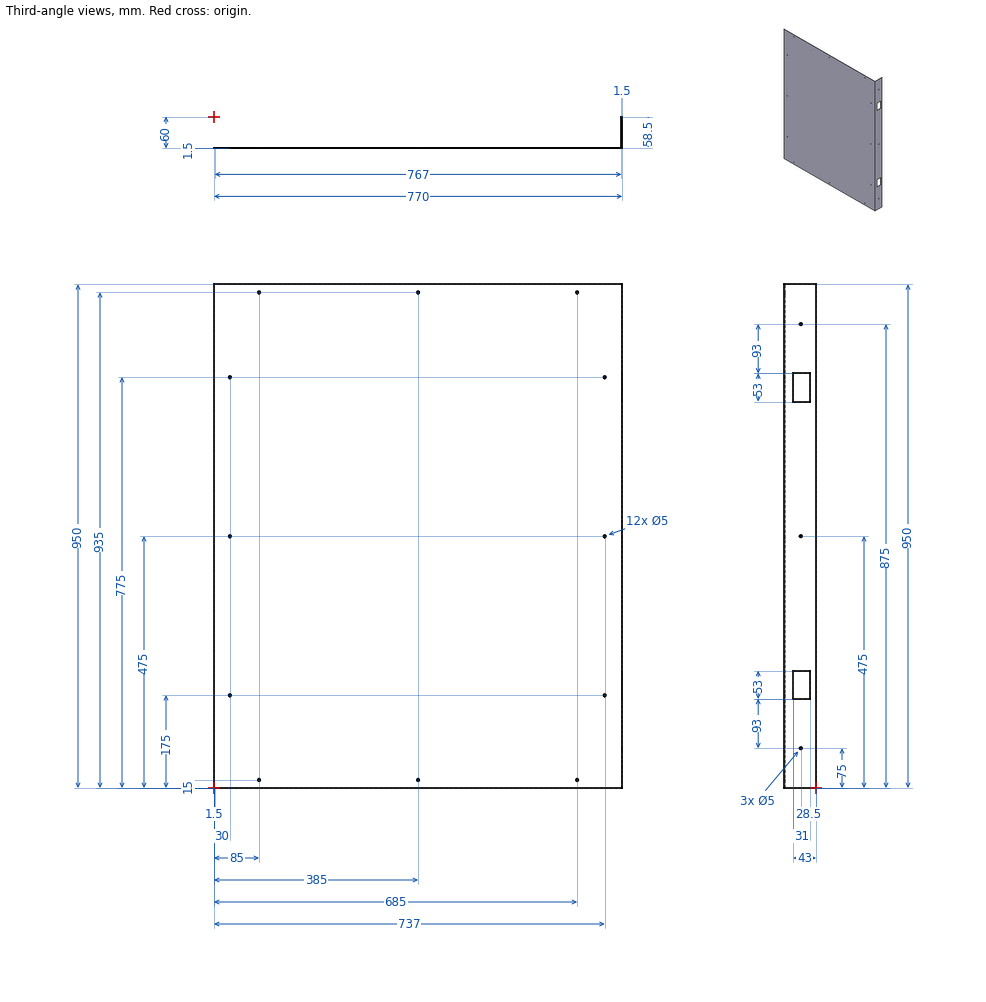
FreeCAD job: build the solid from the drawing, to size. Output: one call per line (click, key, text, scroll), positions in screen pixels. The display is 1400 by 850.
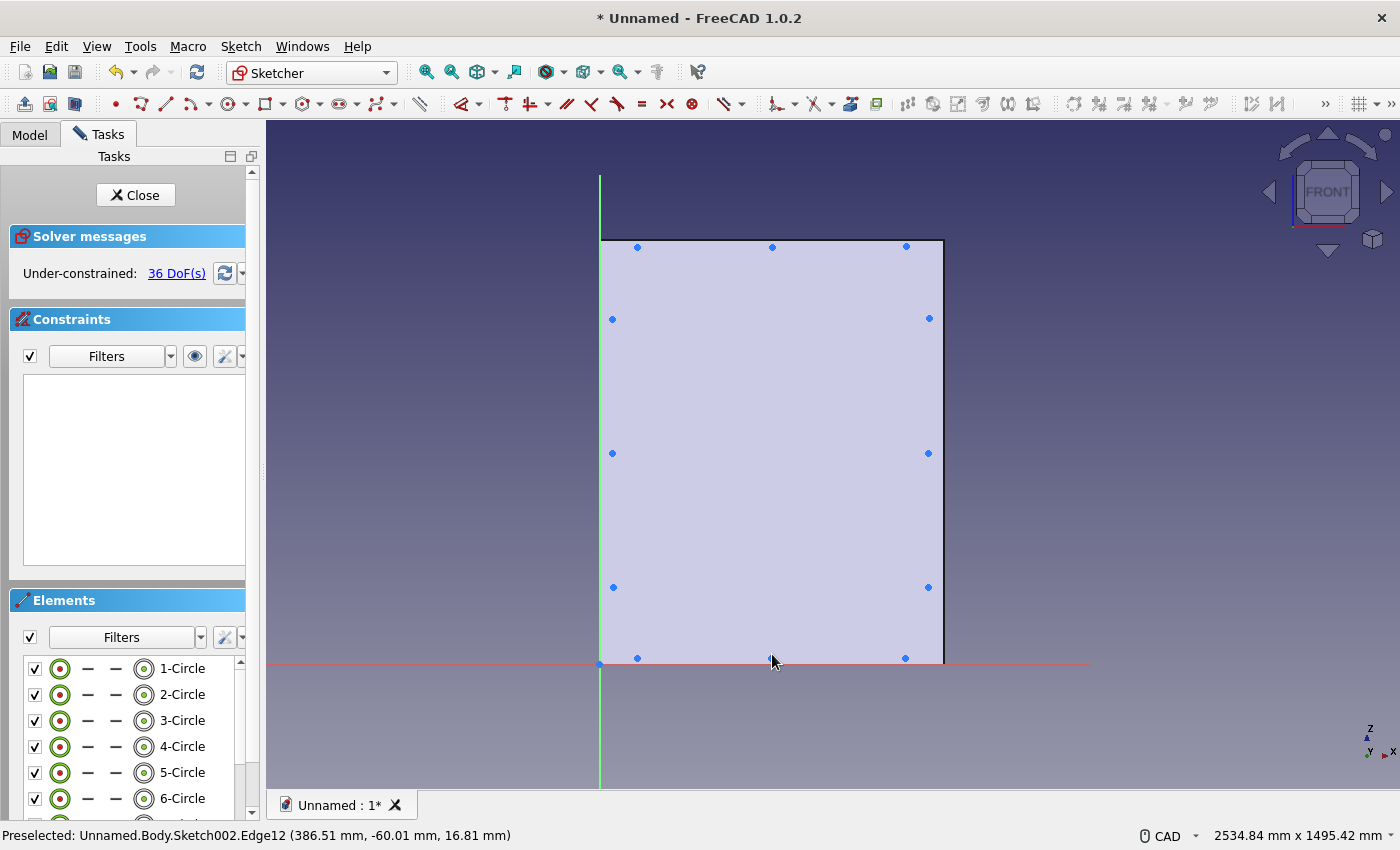
scroll(930, 452, up, 10)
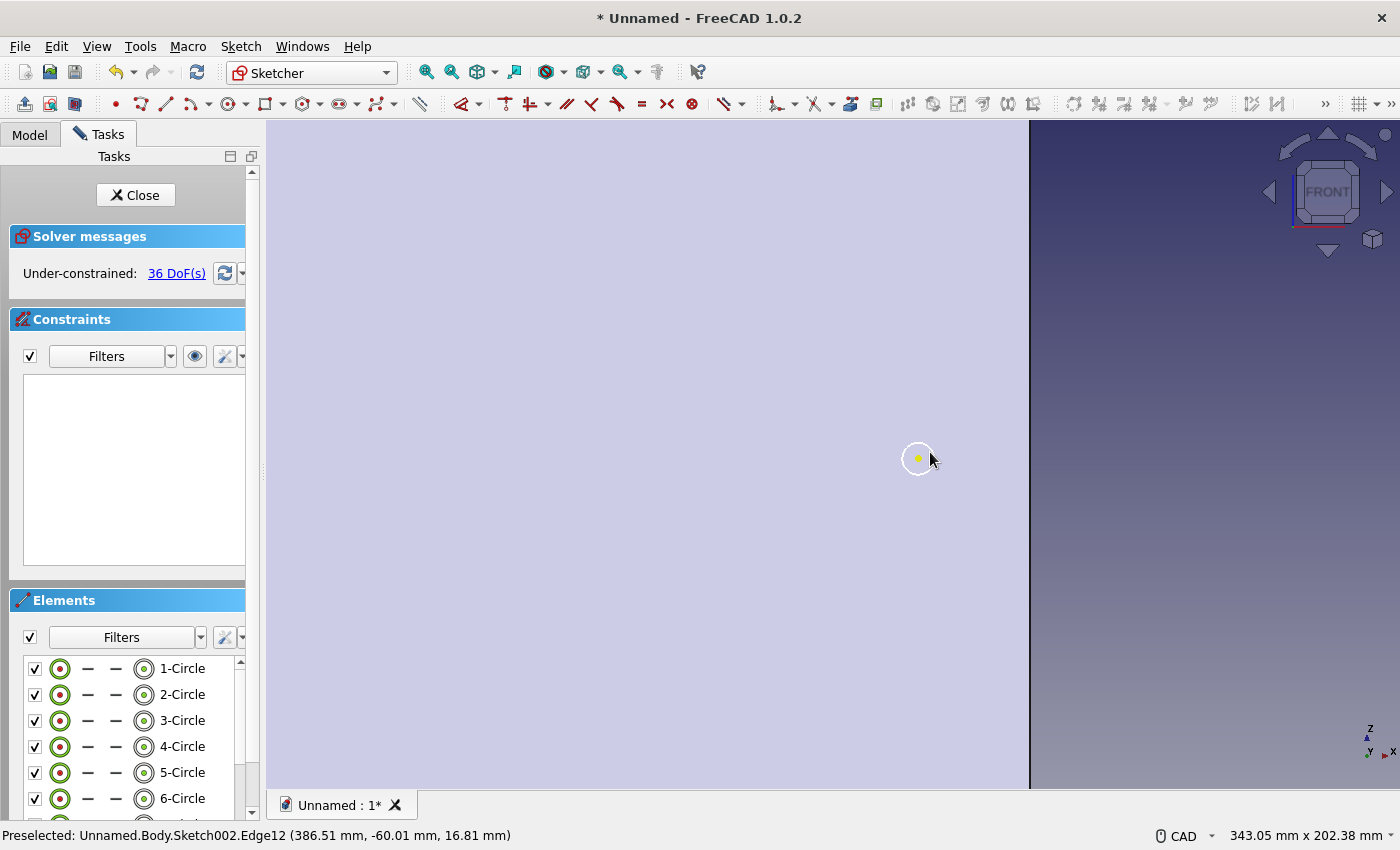
click(930, 447)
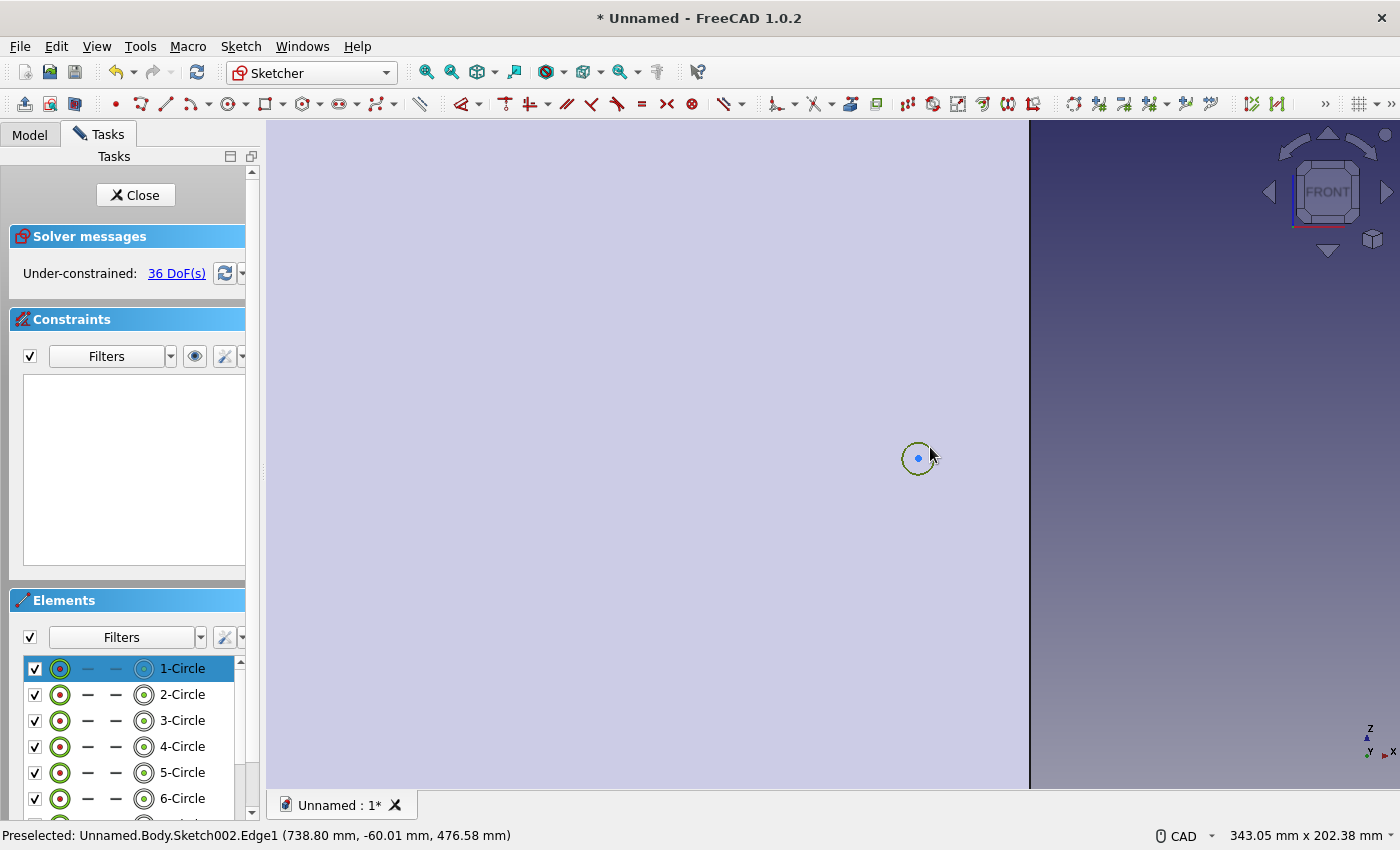
scroll(930, 452, down, 10)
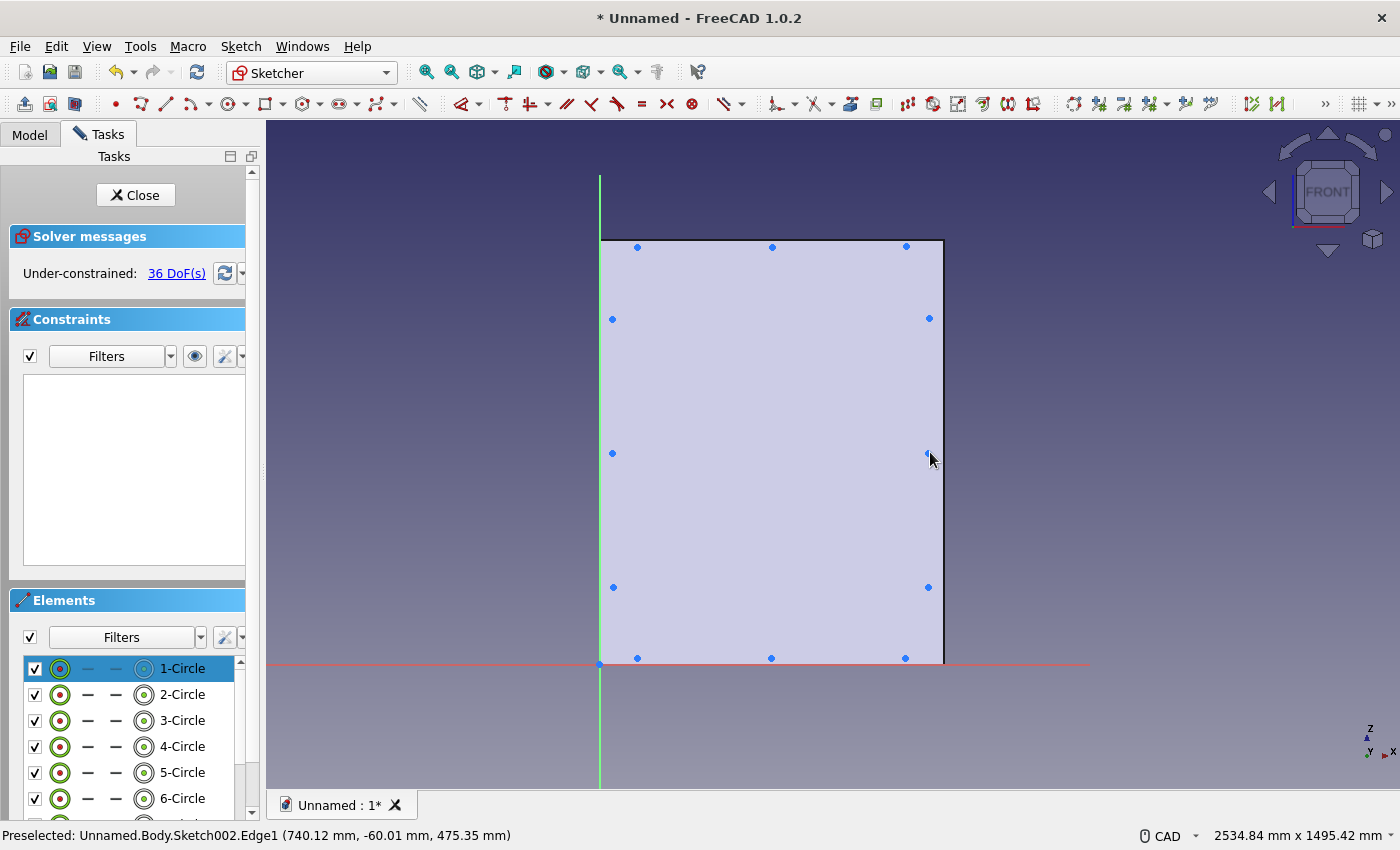
scroll(931, 318, up, 11)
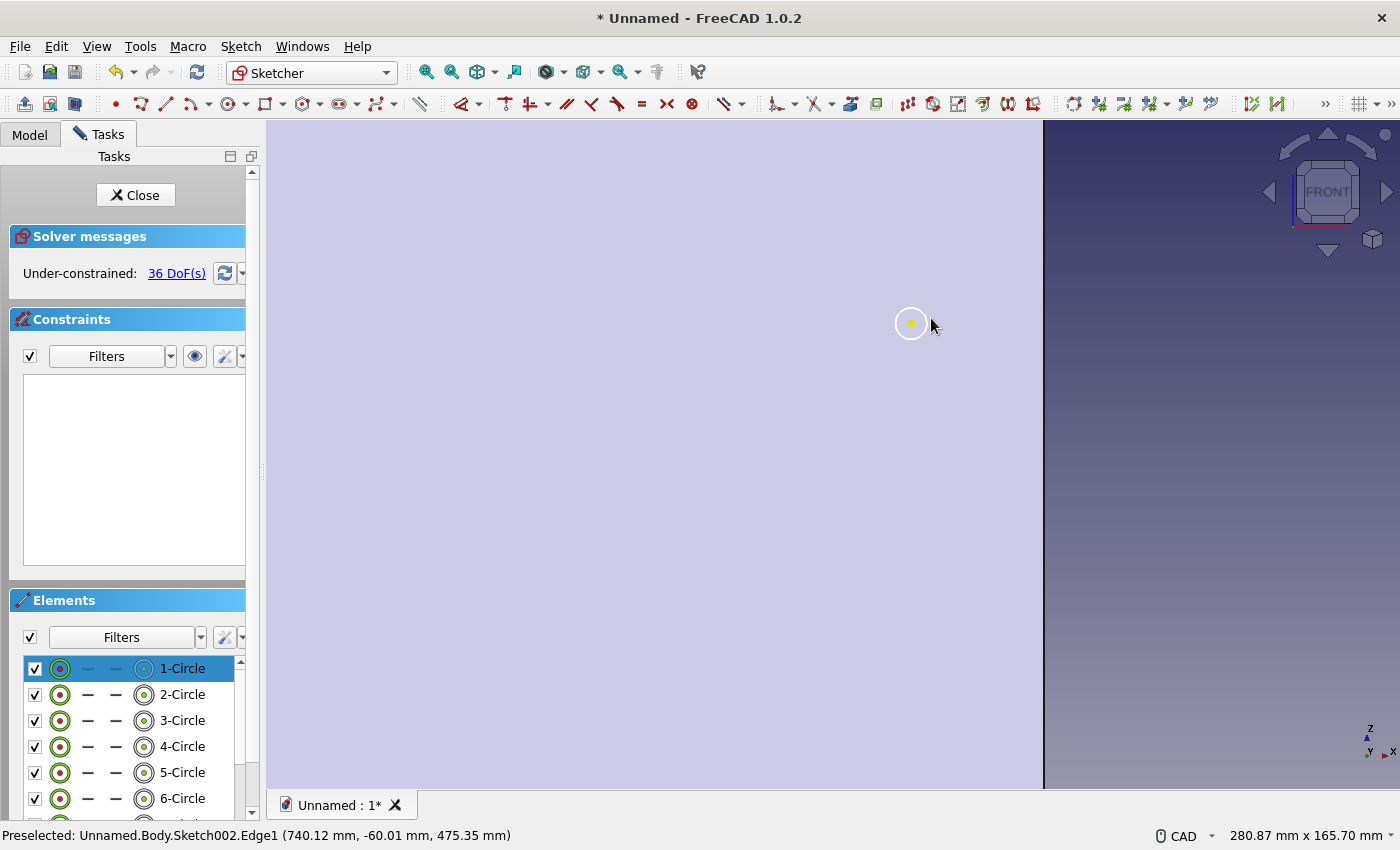
click(922, 312)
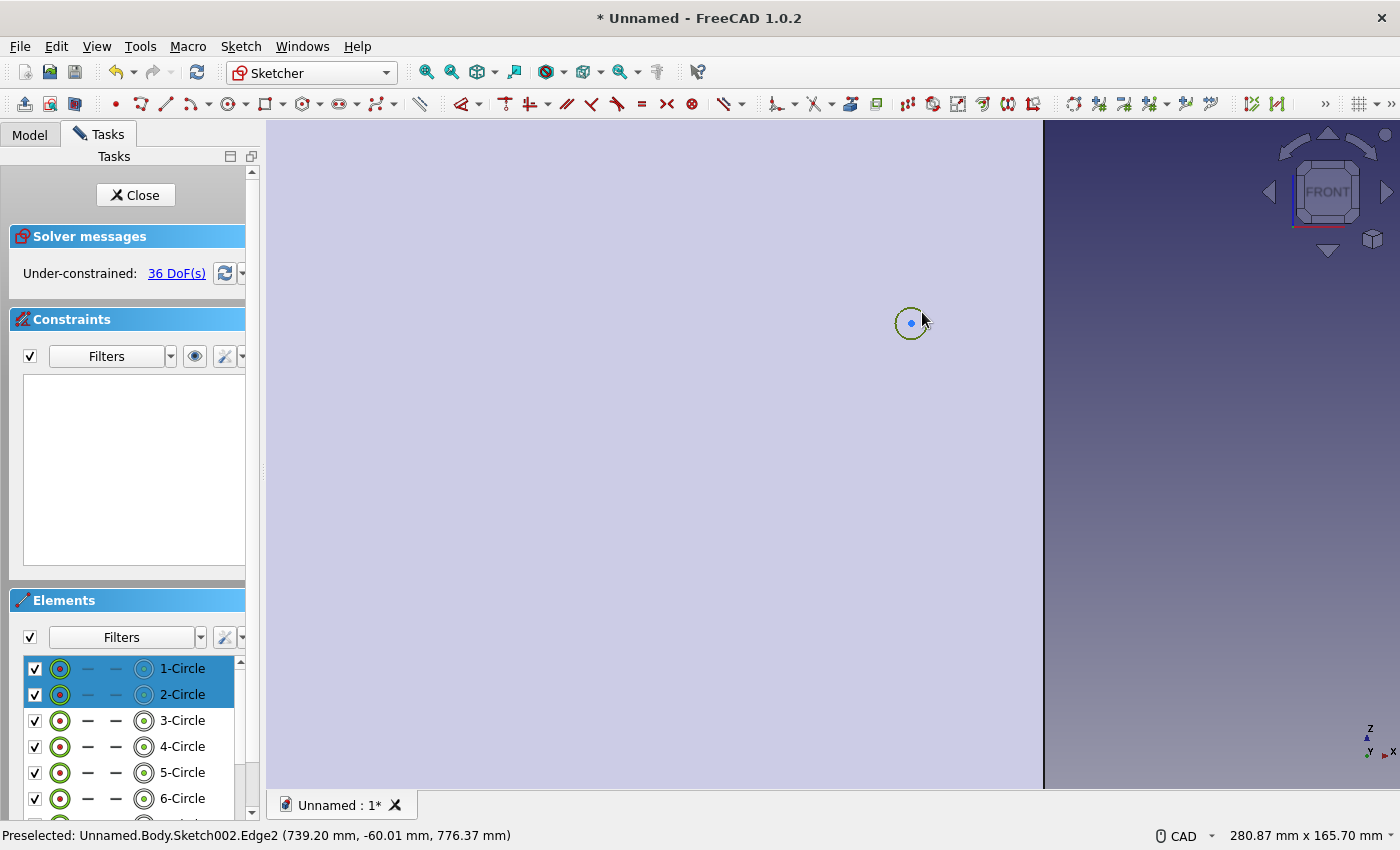
scroll(931, 318, down, 11)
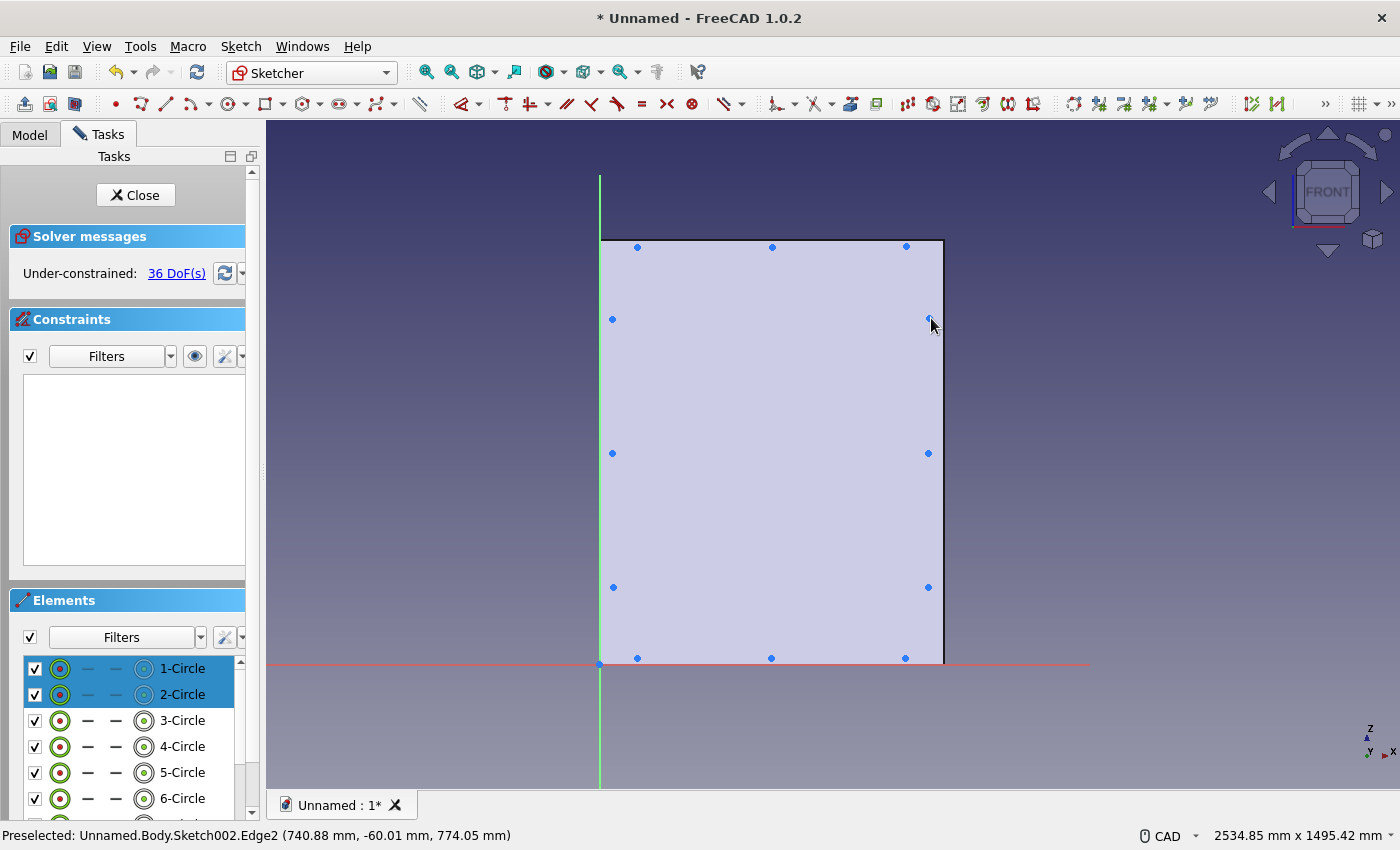
scroll(930, 586, up, 10)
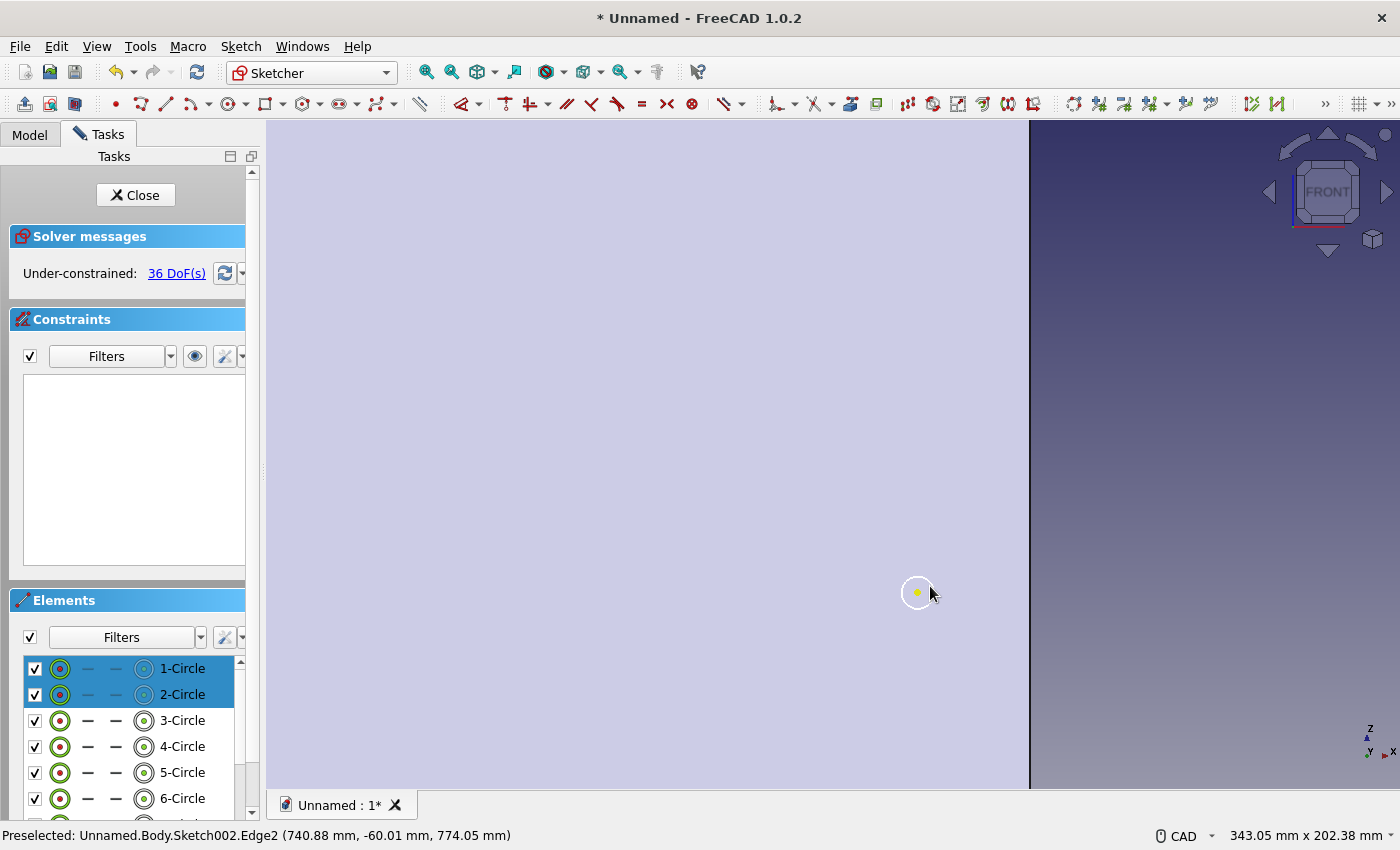
click(929, 581)